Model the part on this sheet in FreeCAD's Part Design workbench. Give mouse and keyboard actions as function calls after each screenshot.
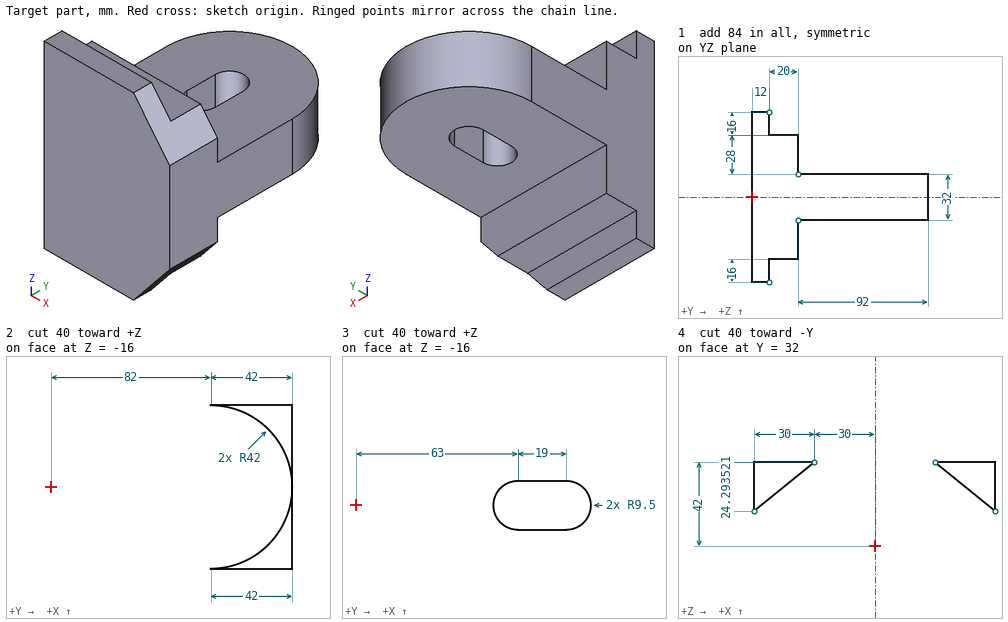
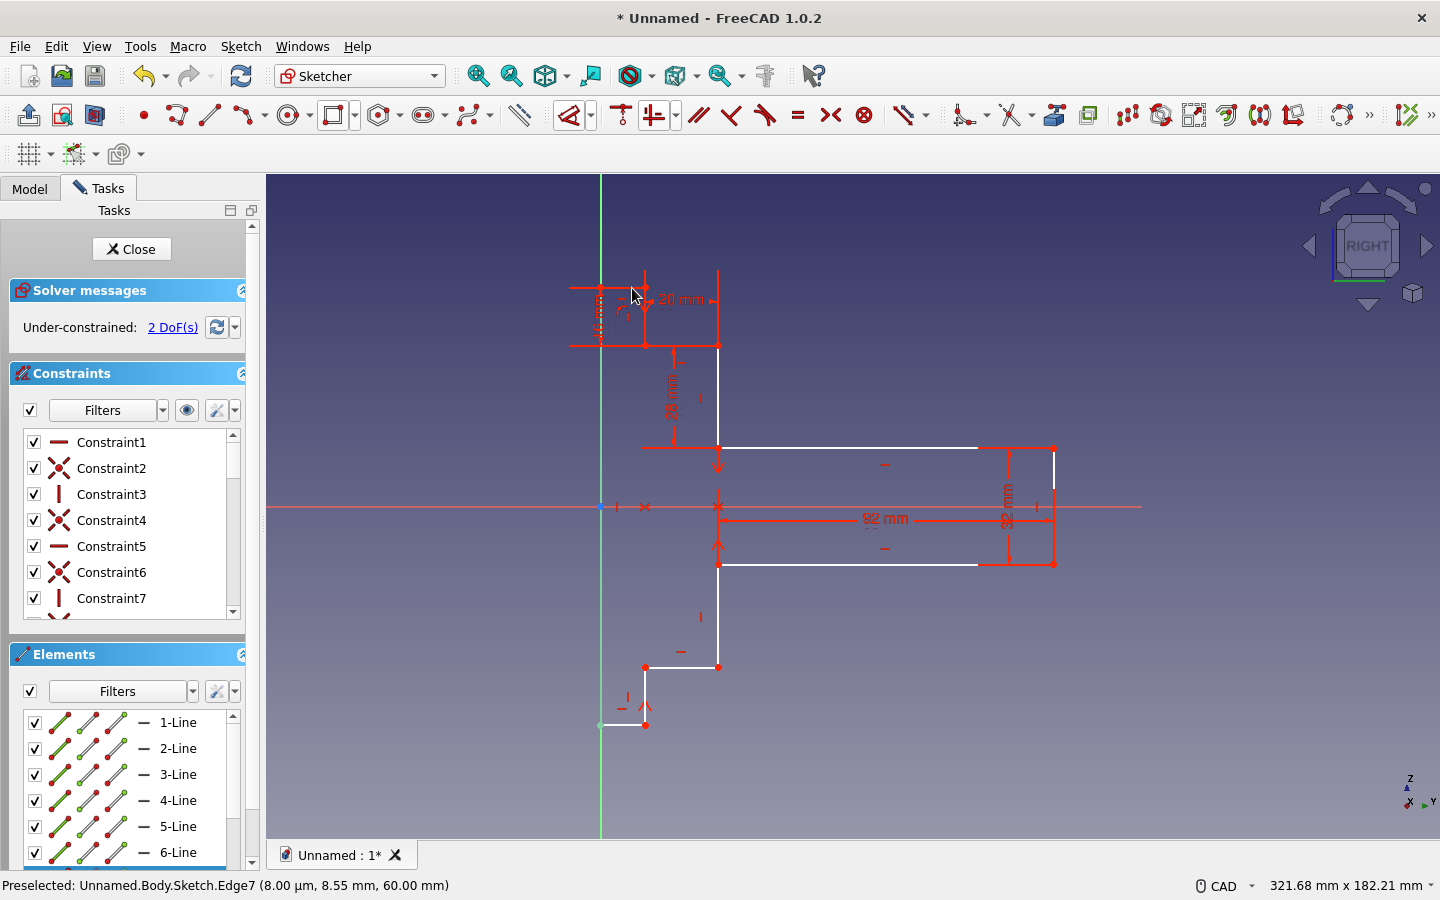
key(l)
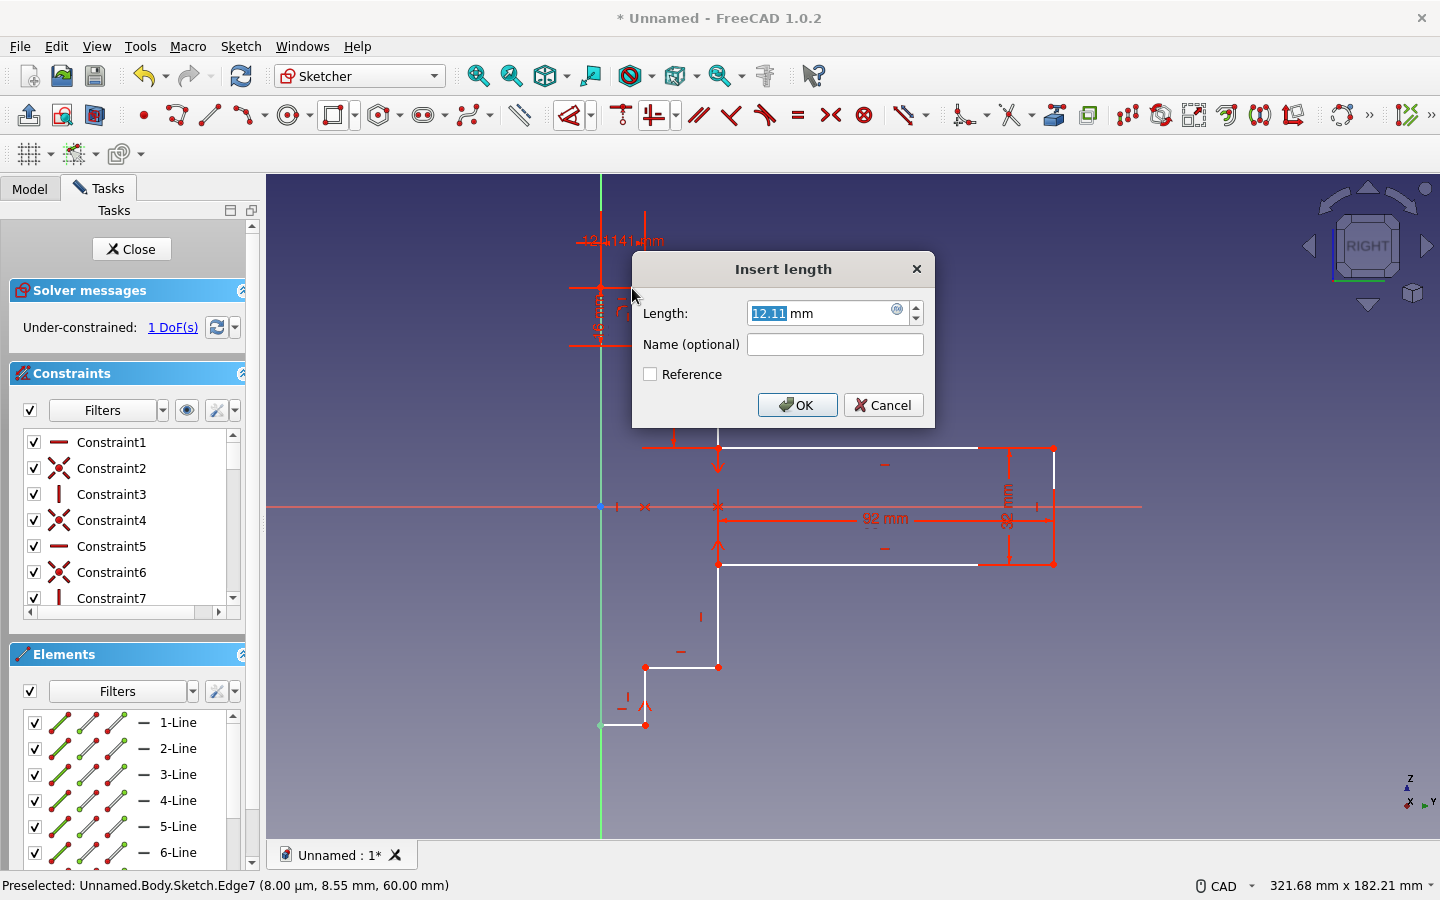
text(12)
key(Return)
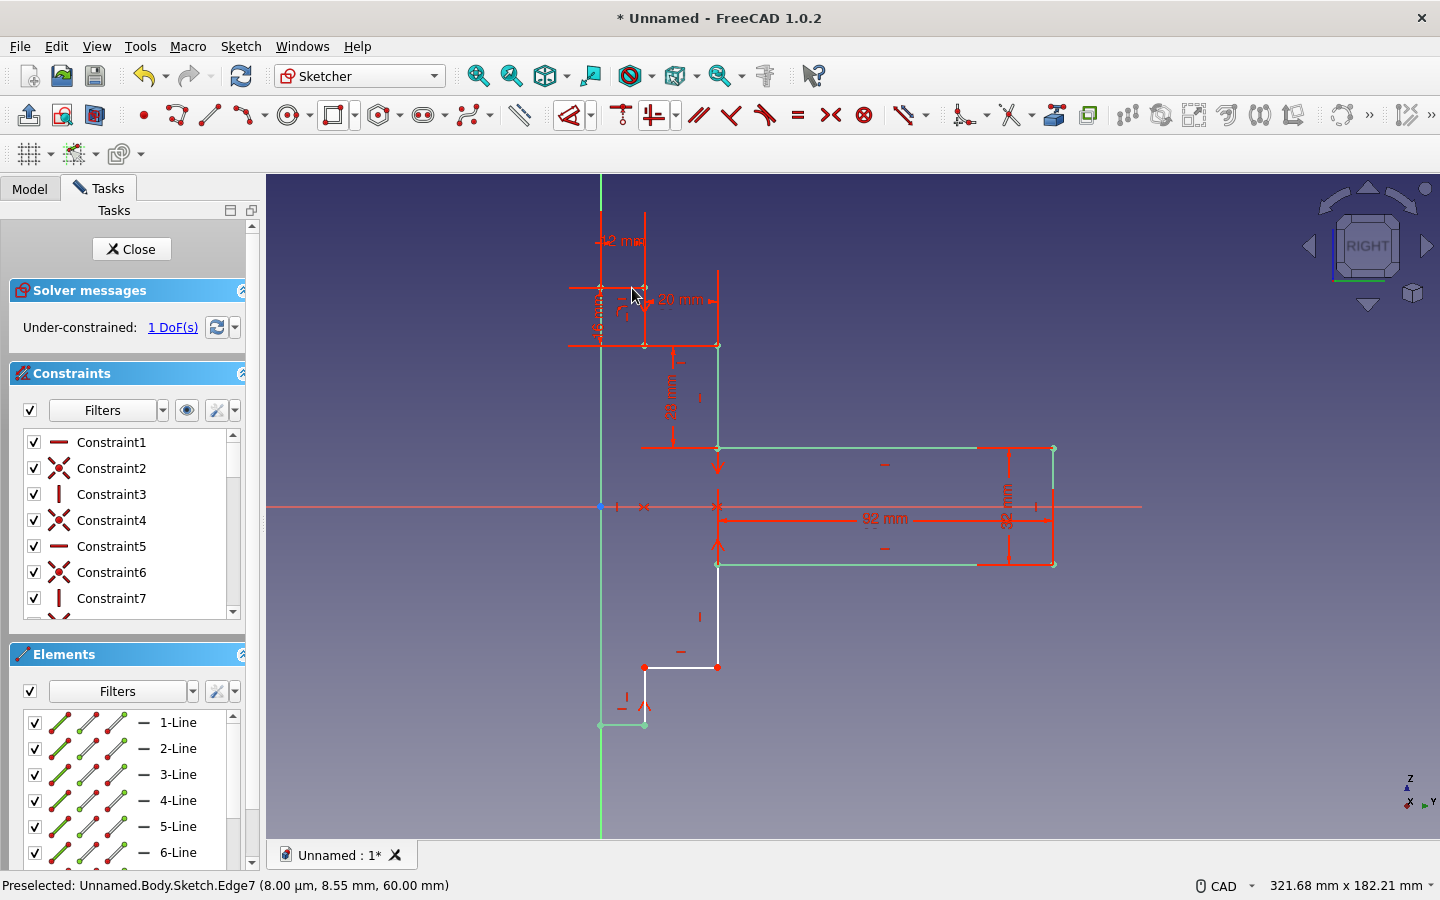
click(645, 708)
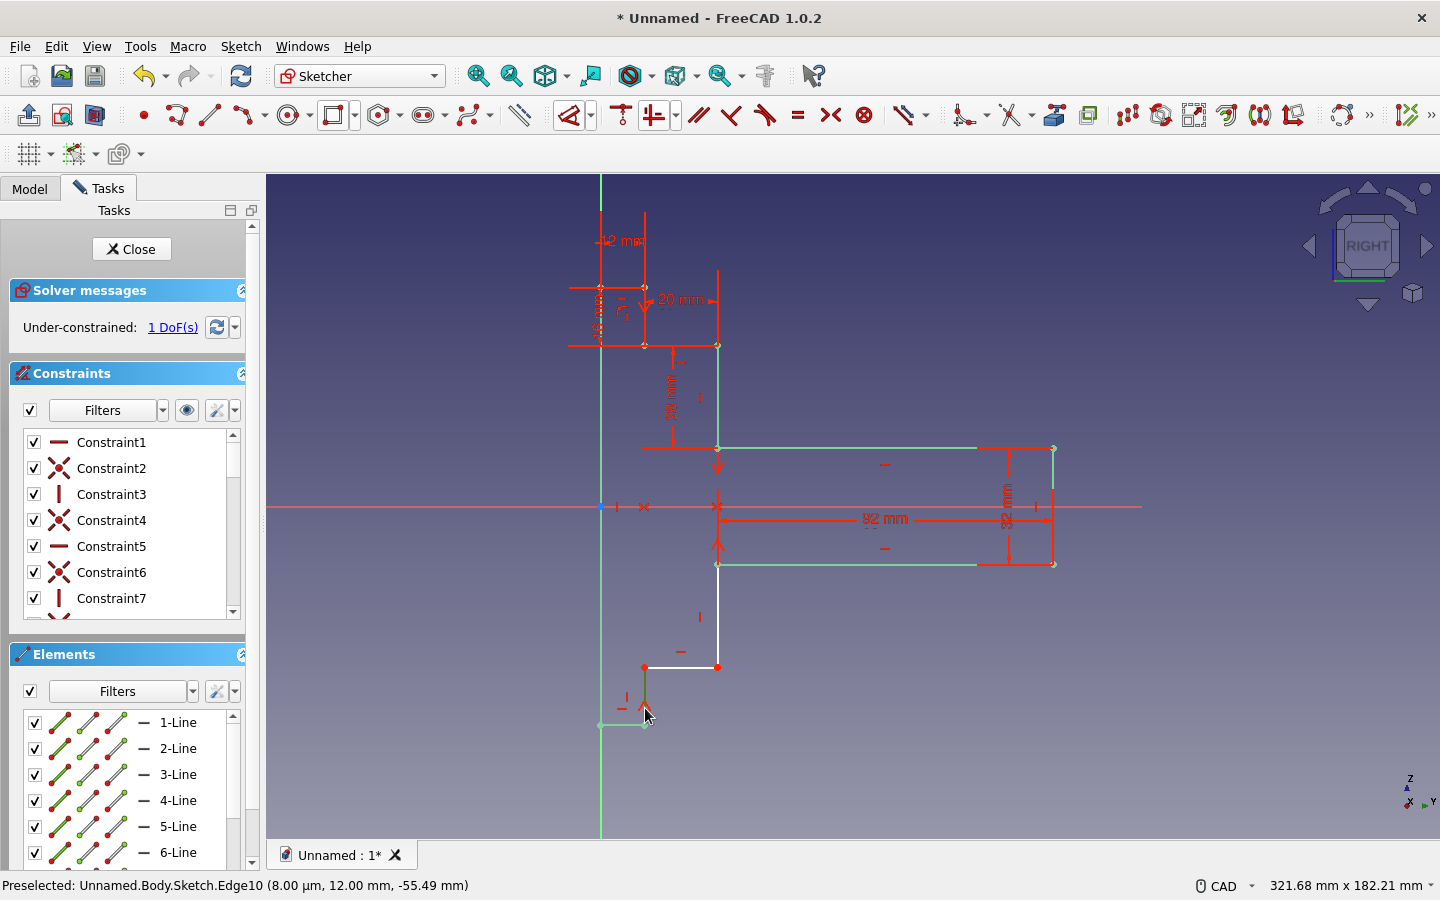
key(i)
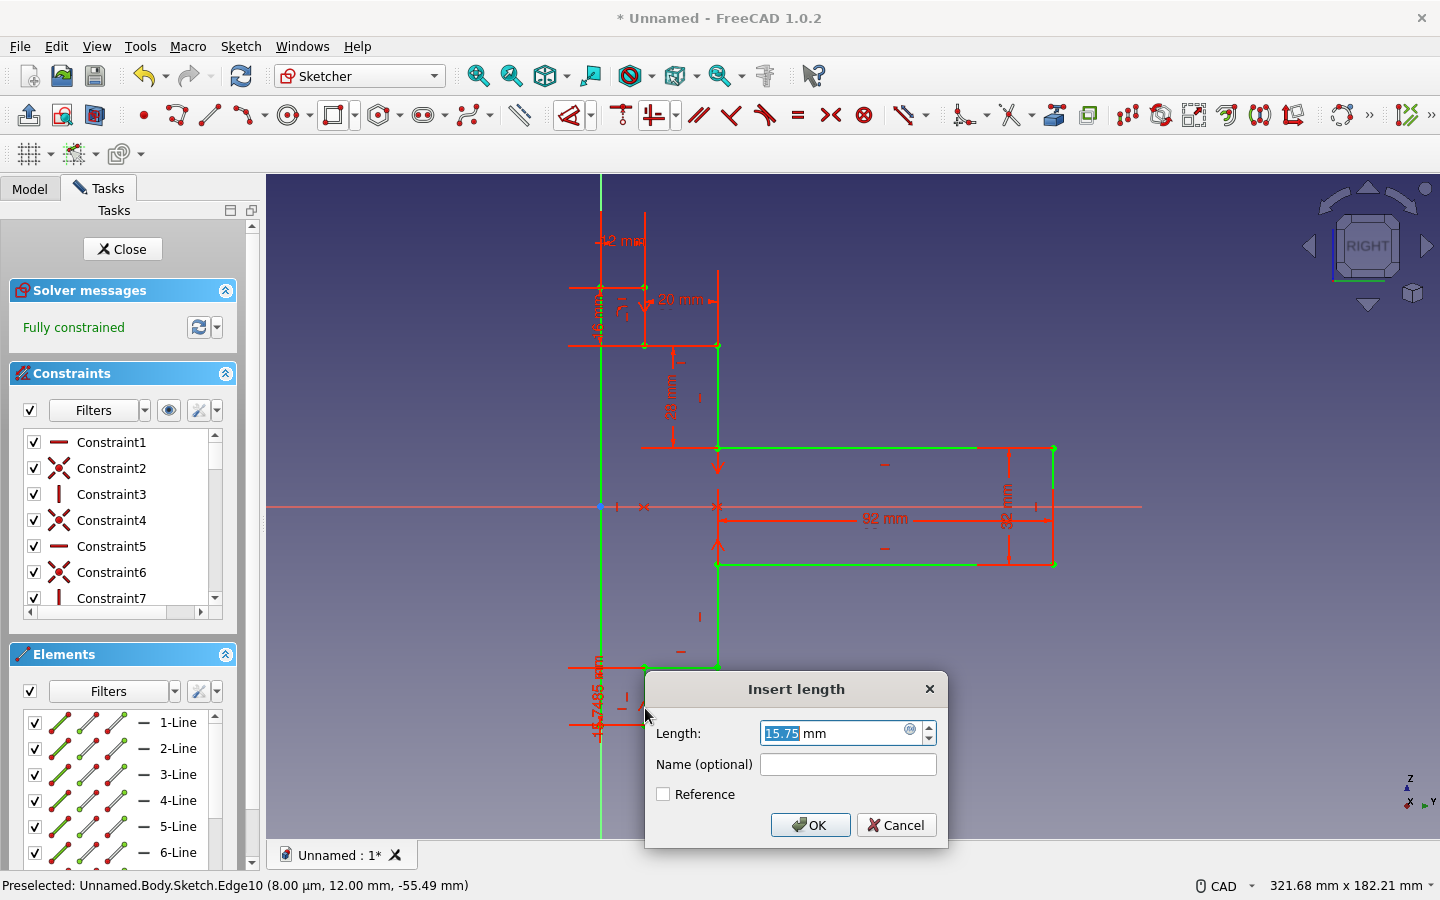
text(16)
key(Return)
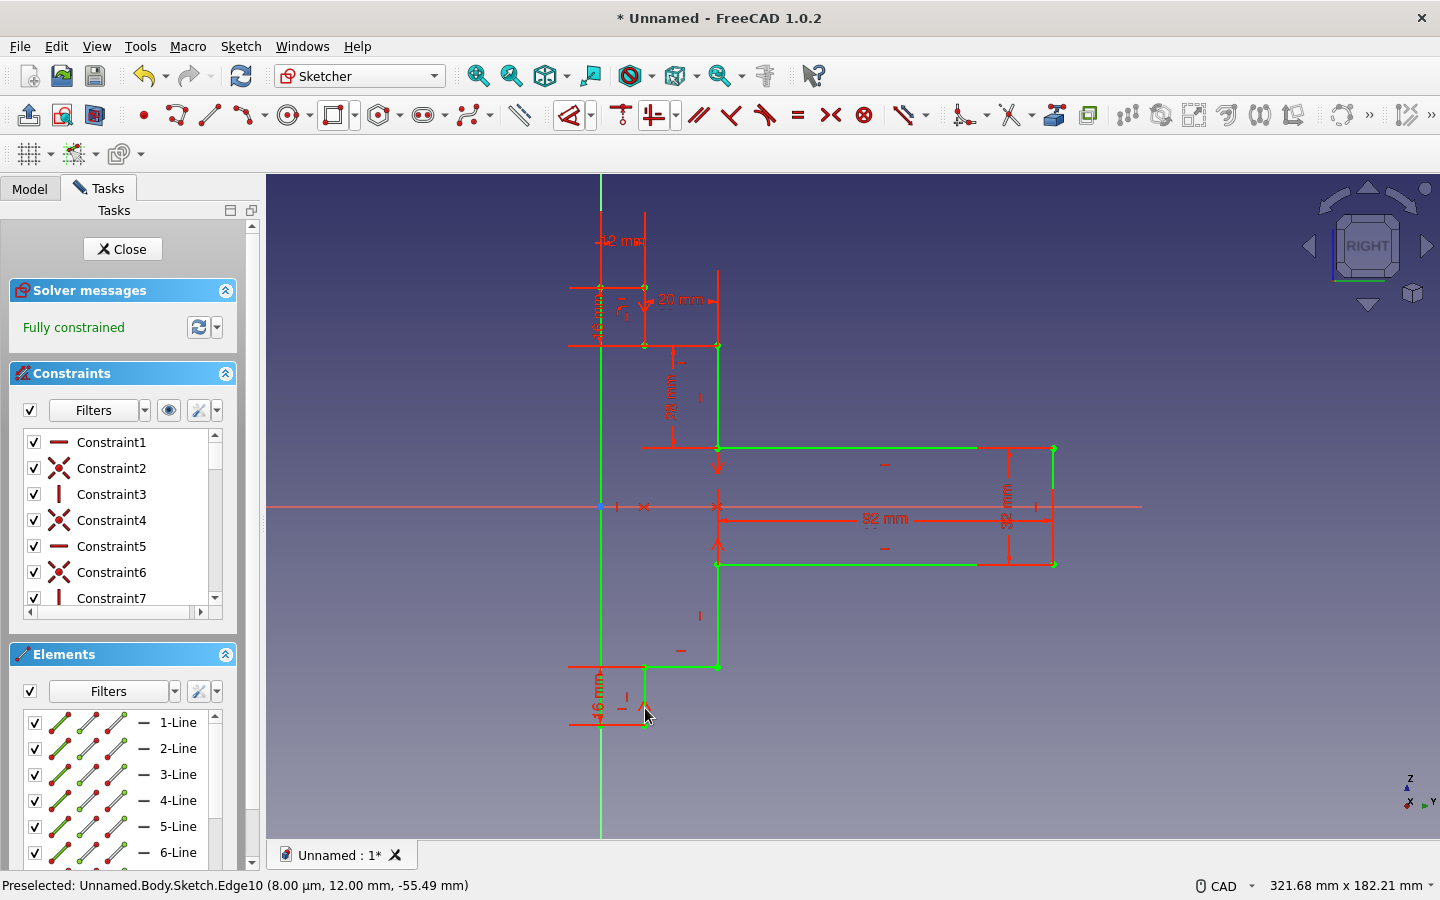
click(123, 249)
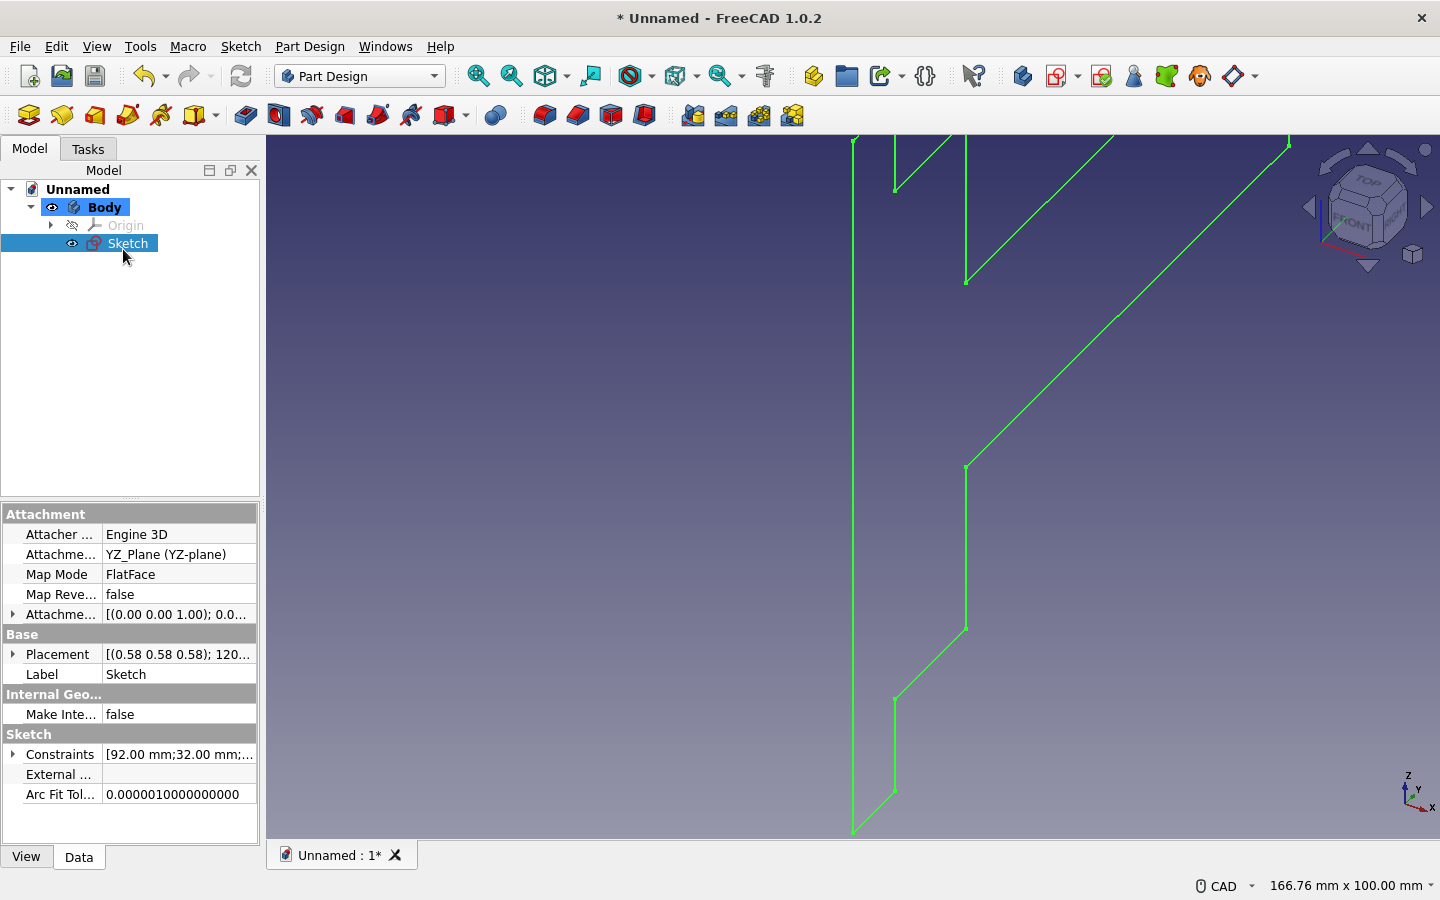
click(29, 116)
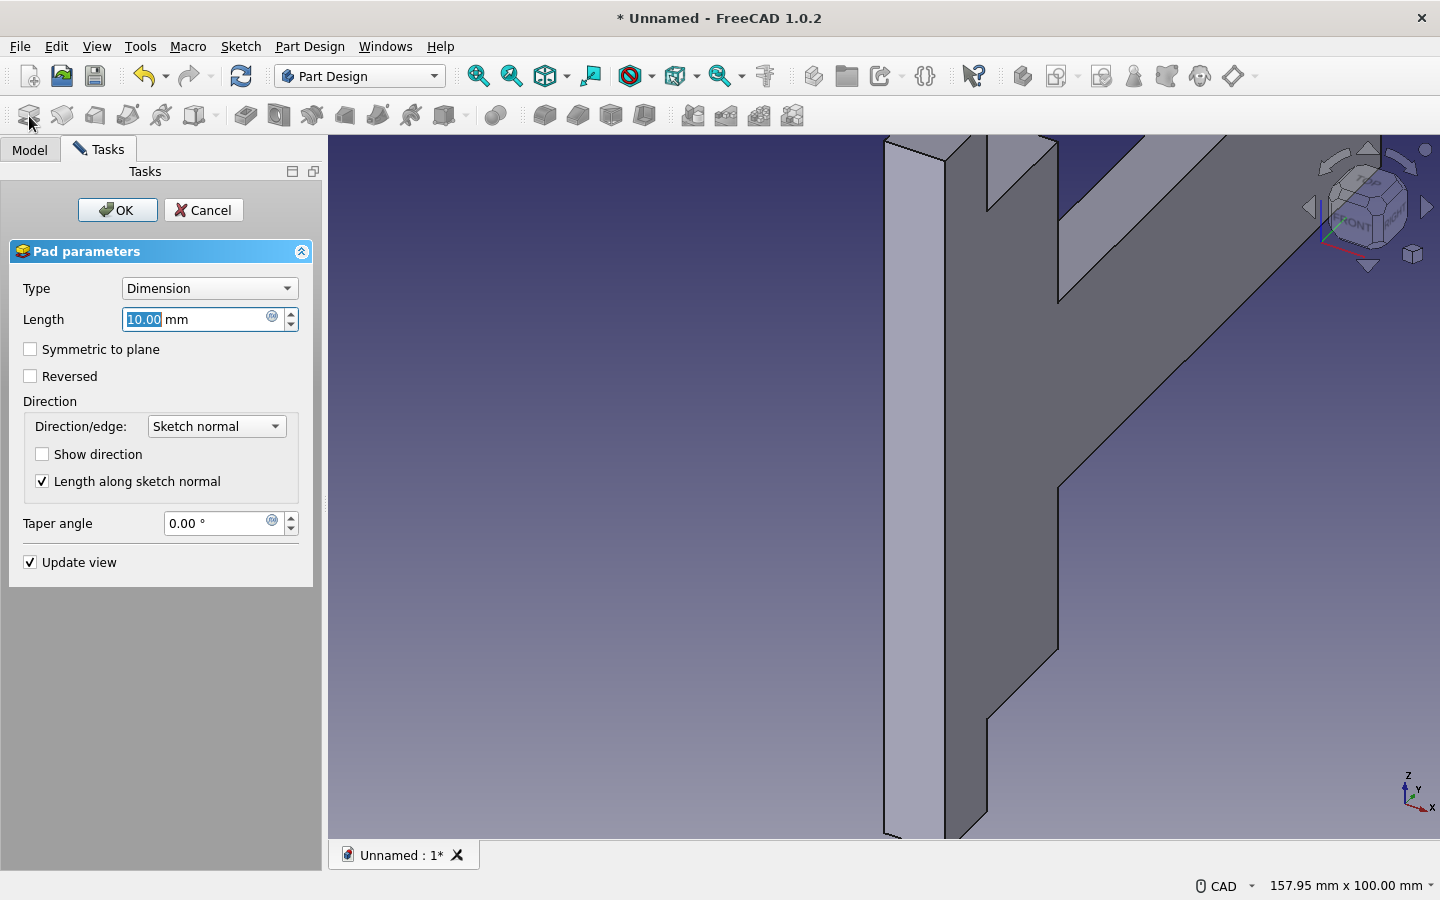
text(84)
key(Tab)